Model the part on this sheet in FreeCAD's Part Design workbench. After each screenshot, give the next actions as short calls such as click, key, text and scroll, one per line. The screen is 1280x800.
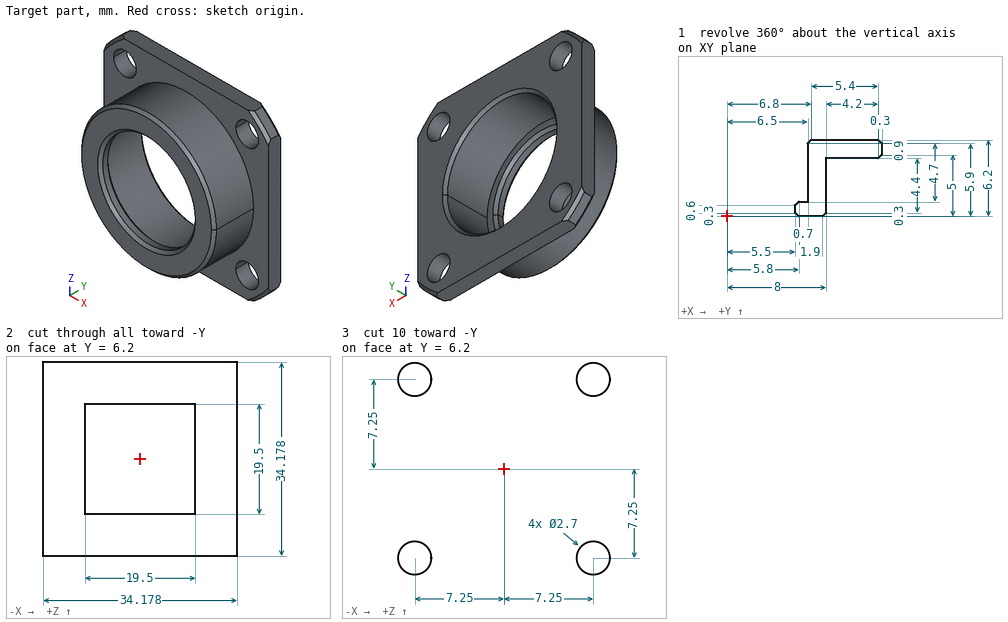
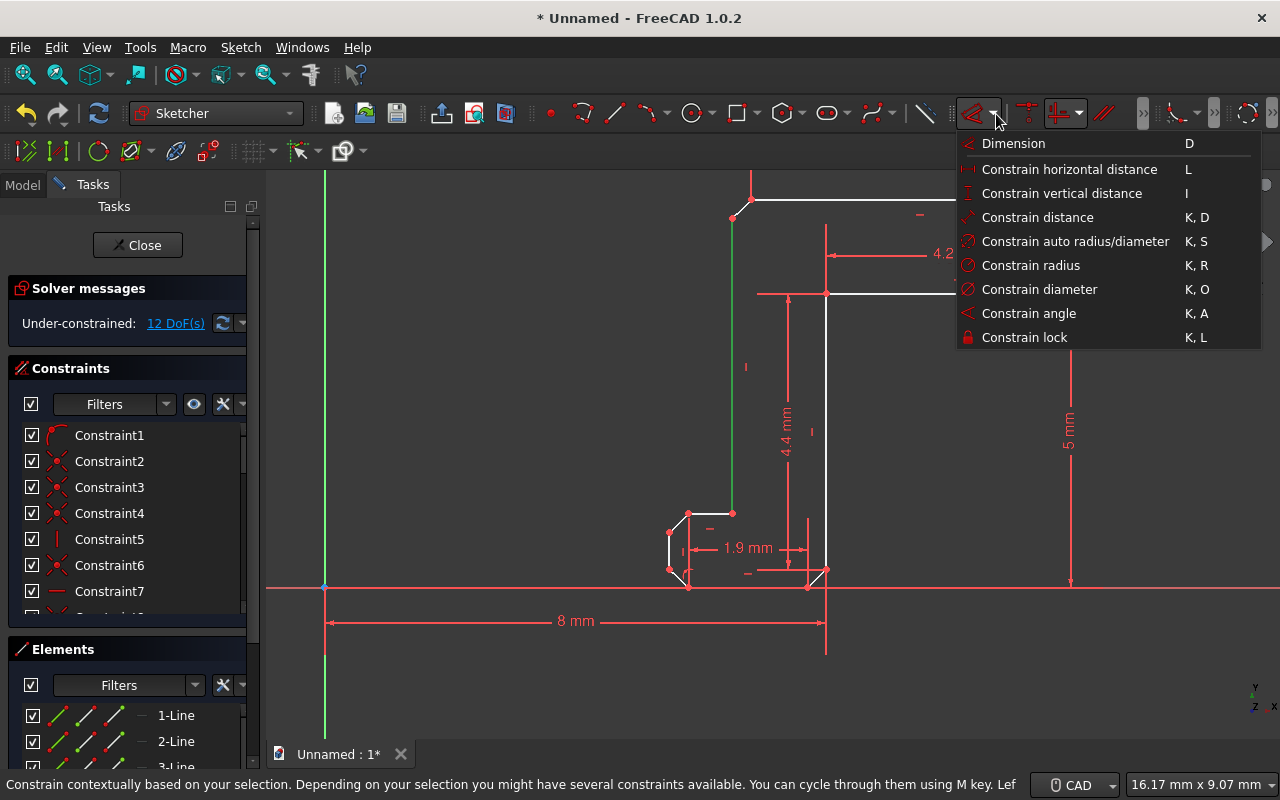
click(1109, 193)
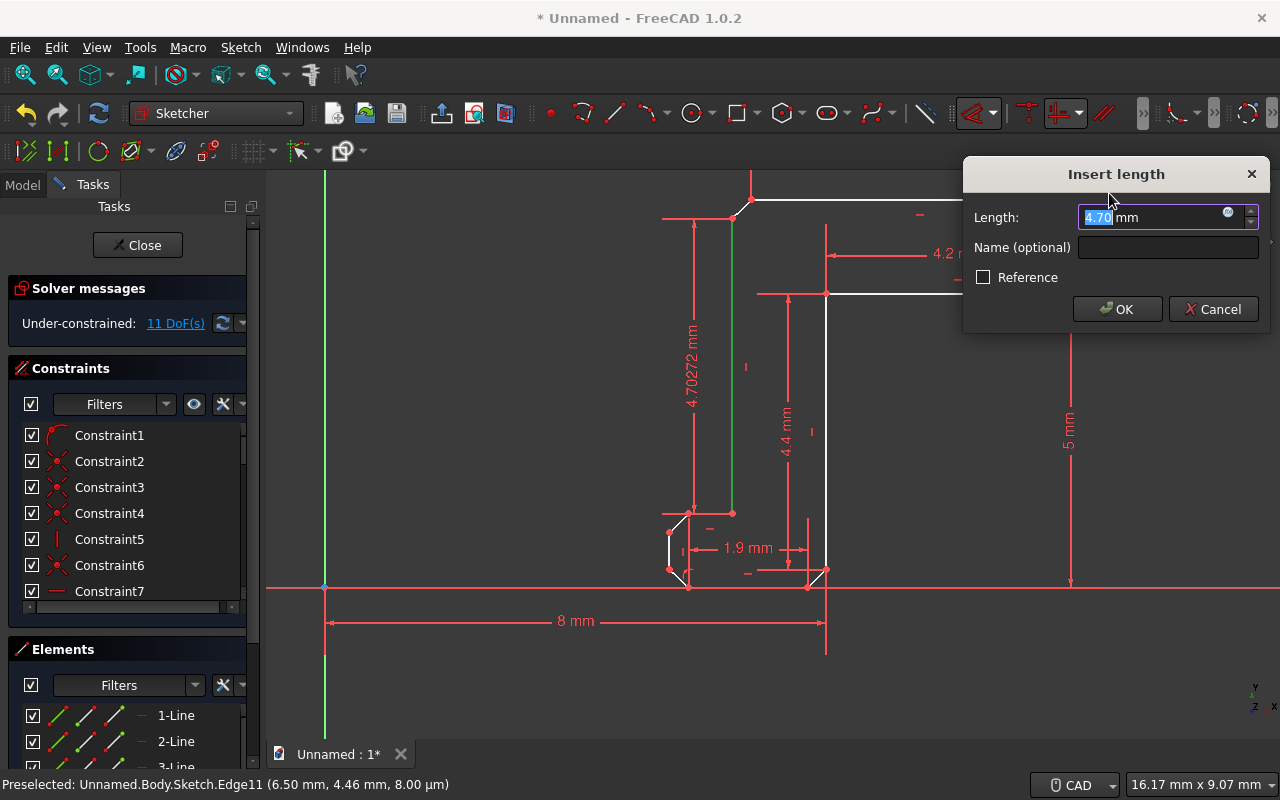
text(4.7)
key(Return)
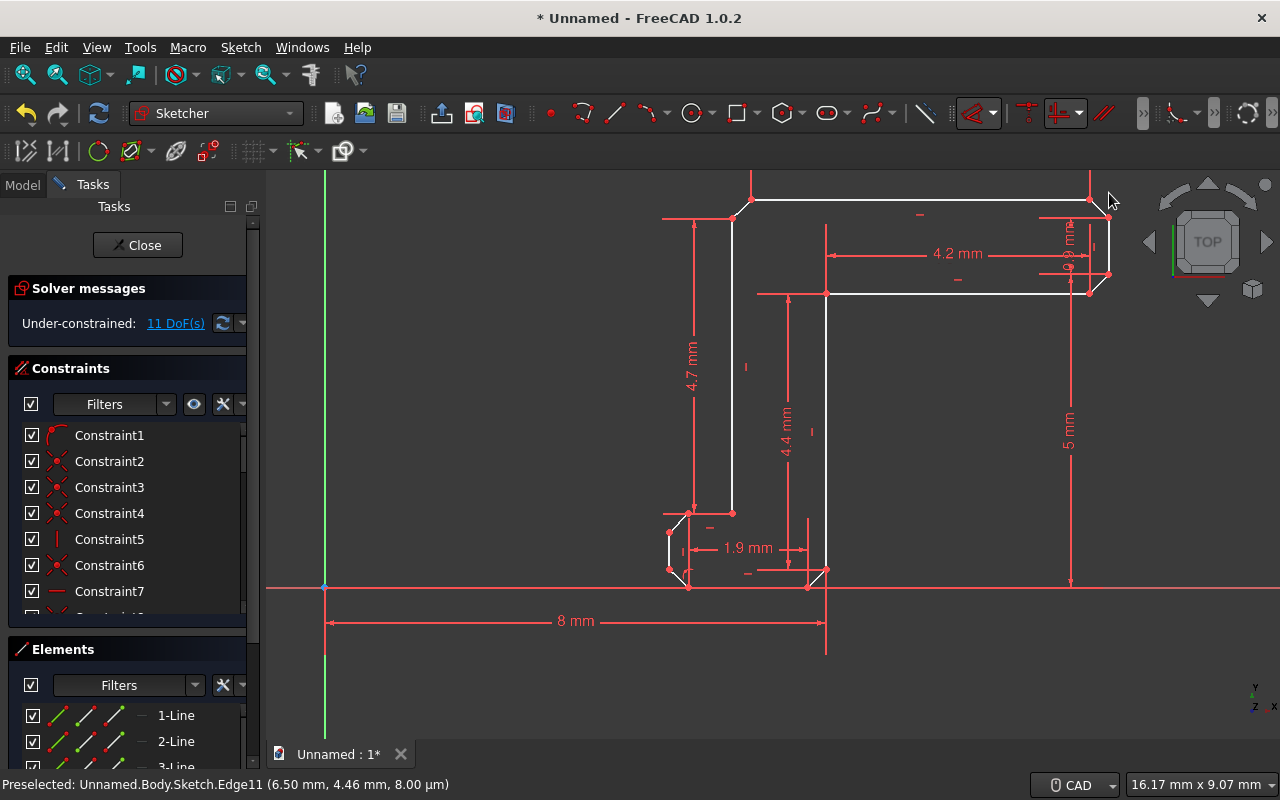
click(719, 514)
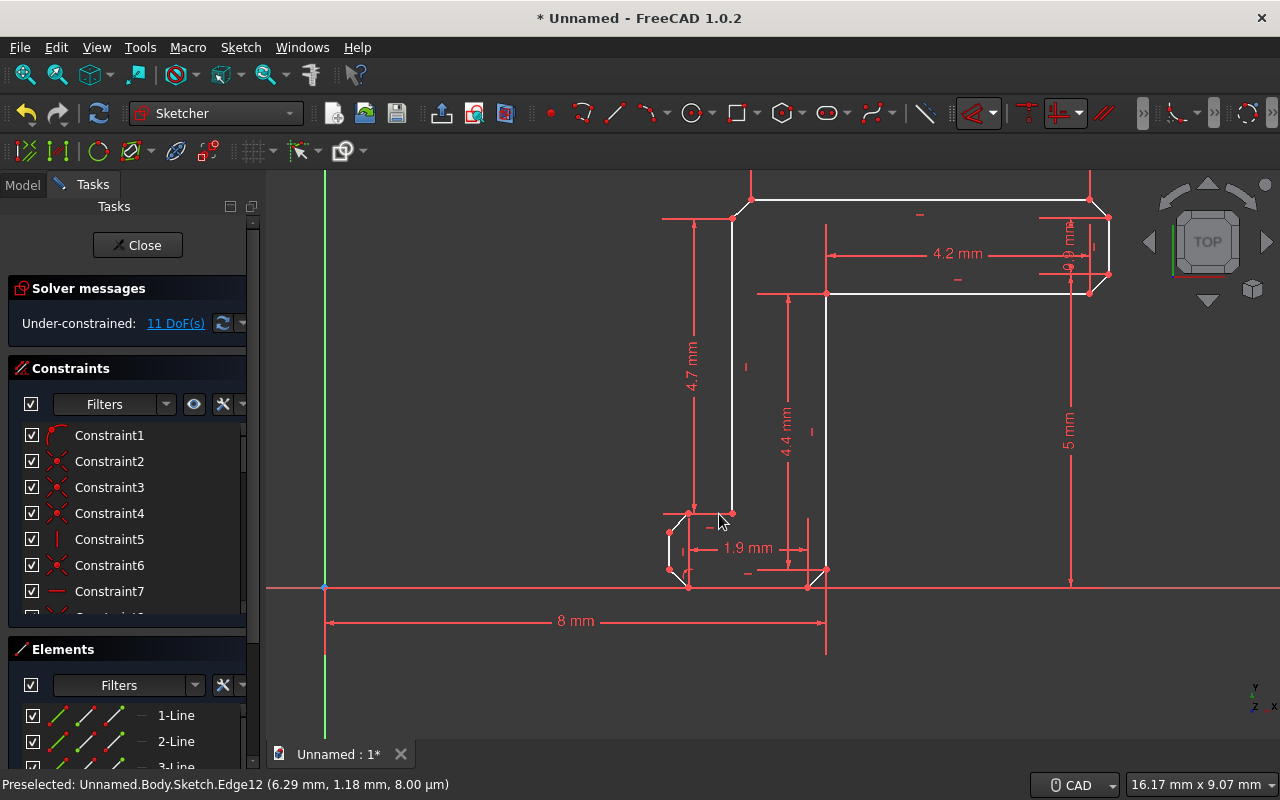
click(996, 114)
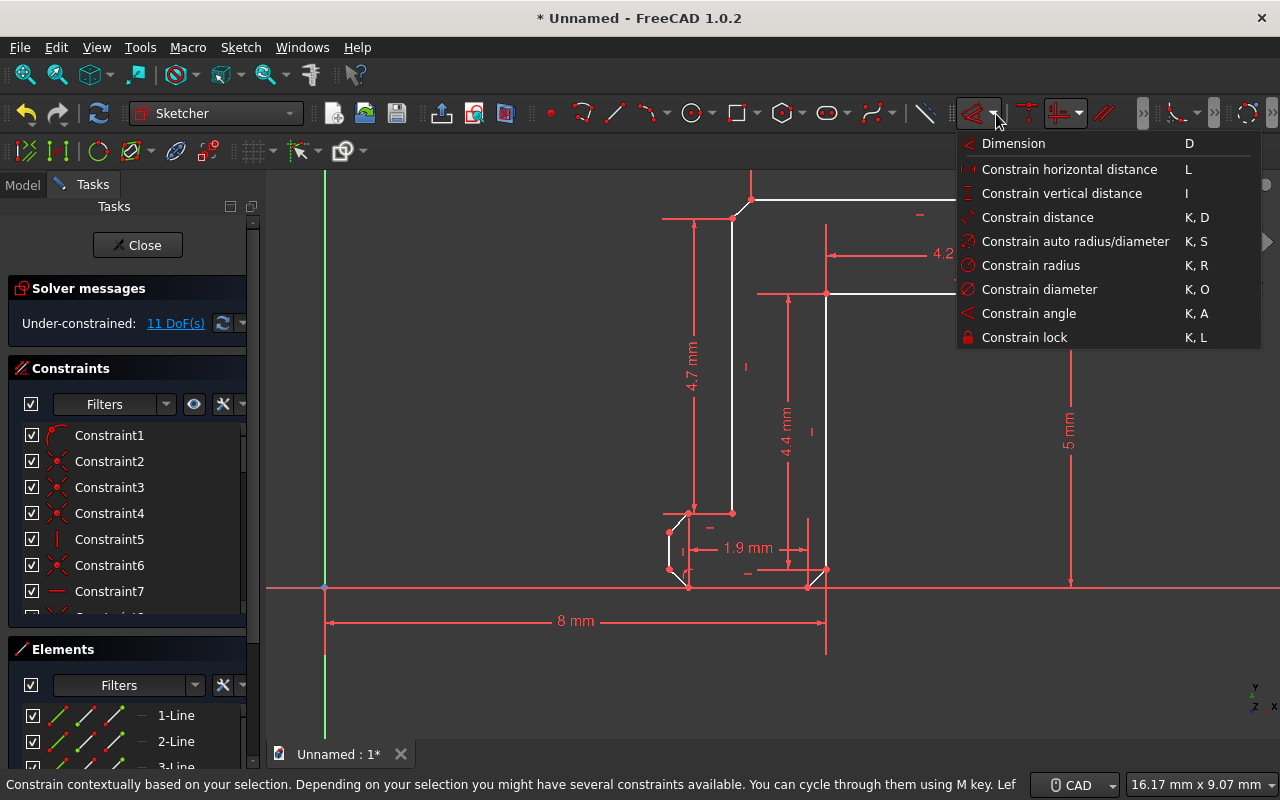
click(1109, 169)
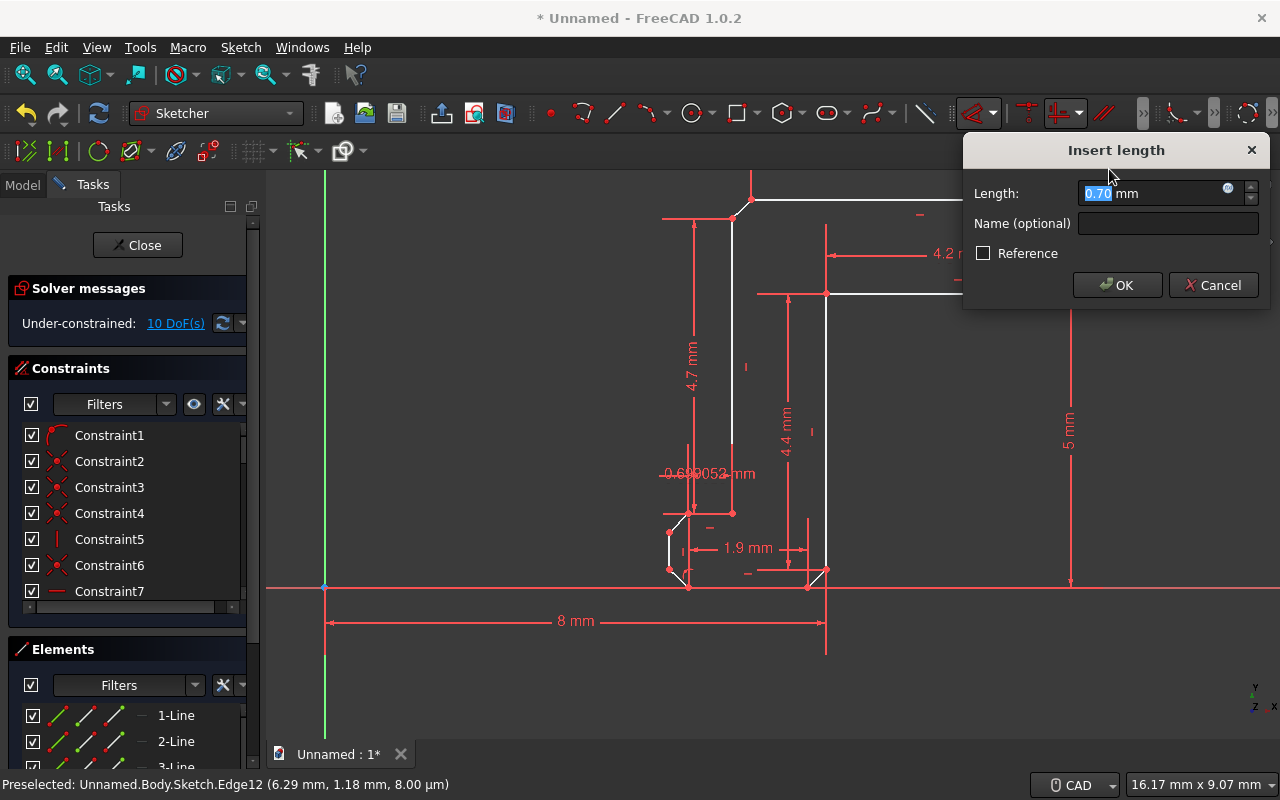
text(0.7)
key(Return)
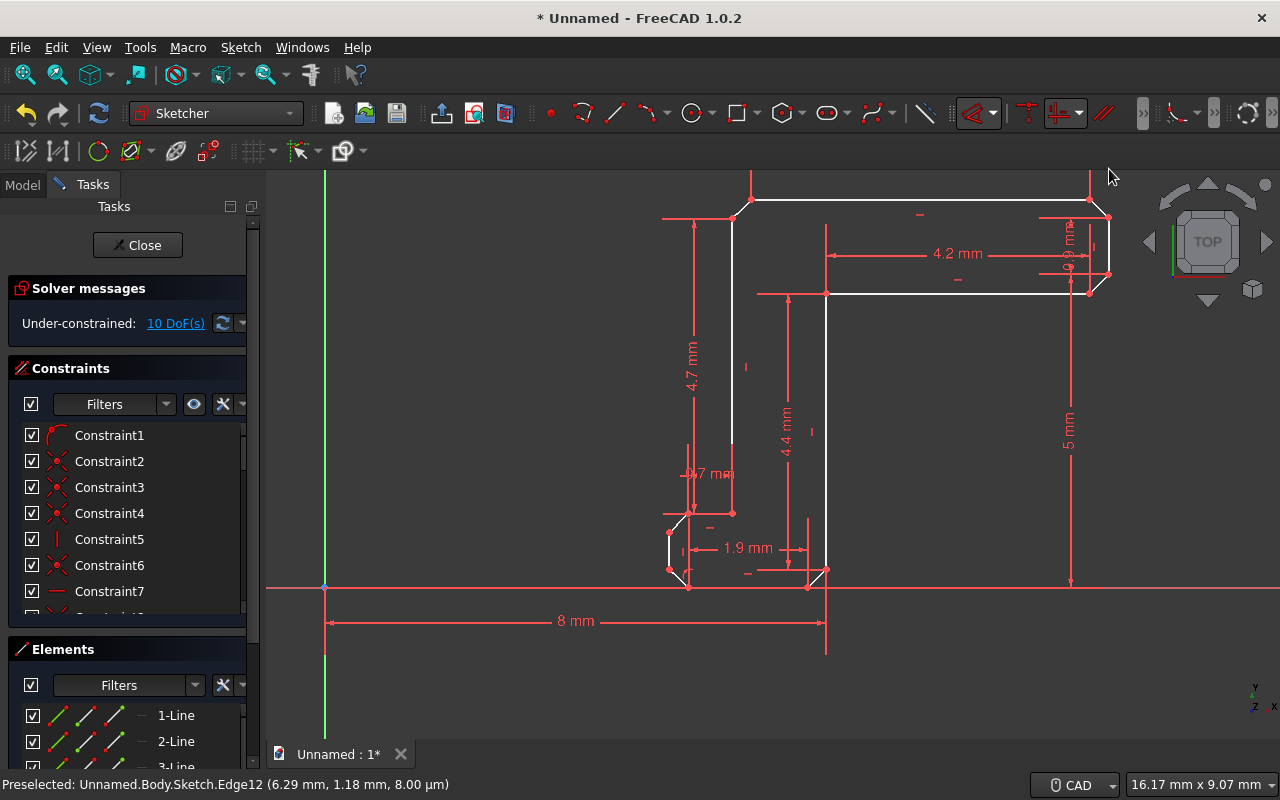
scroll(669, 544, up, 2)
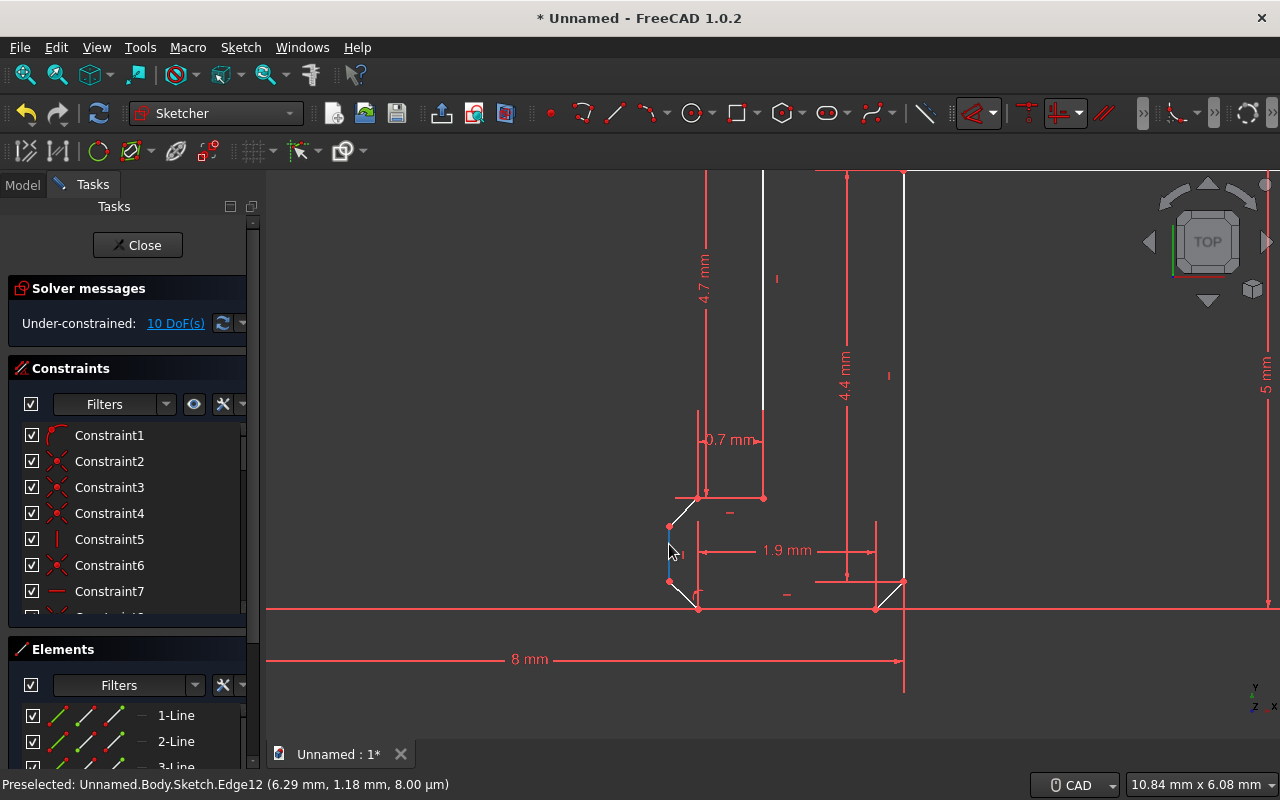
click(669, 543)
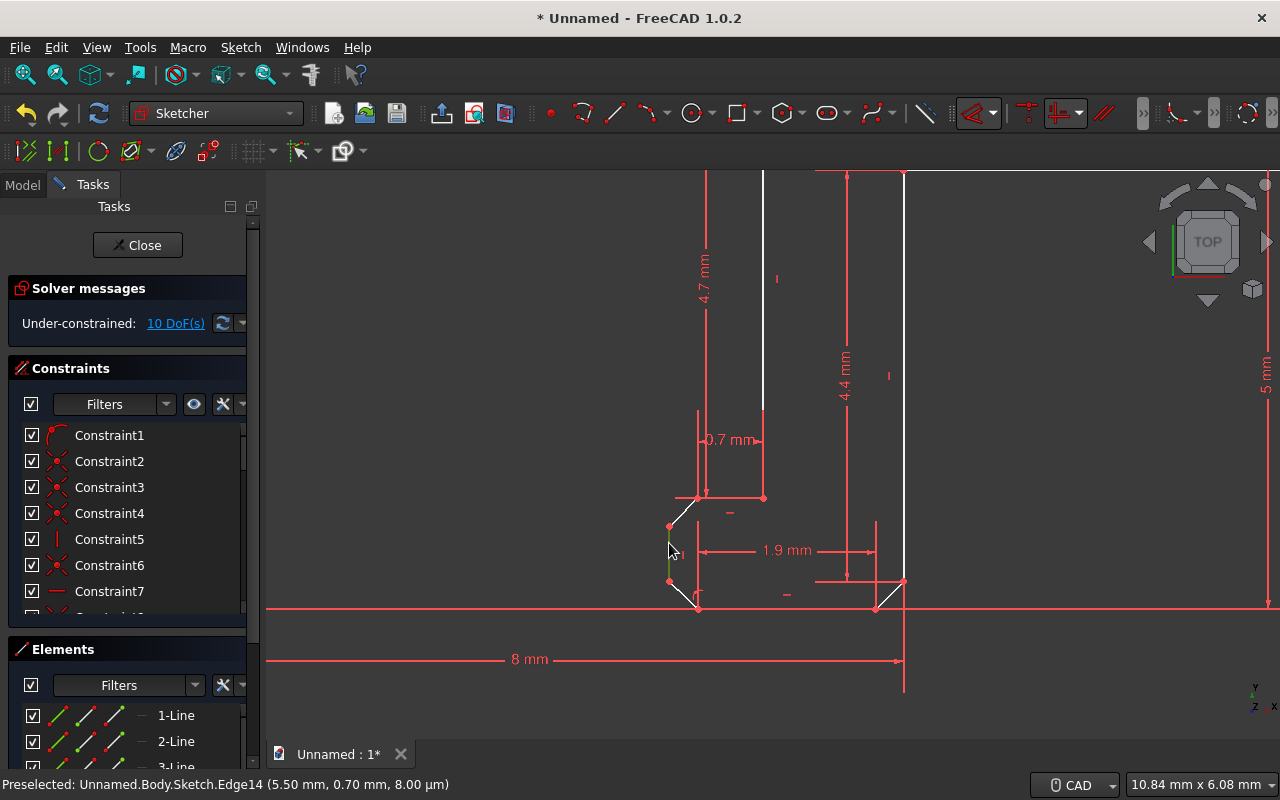
click(996, 114)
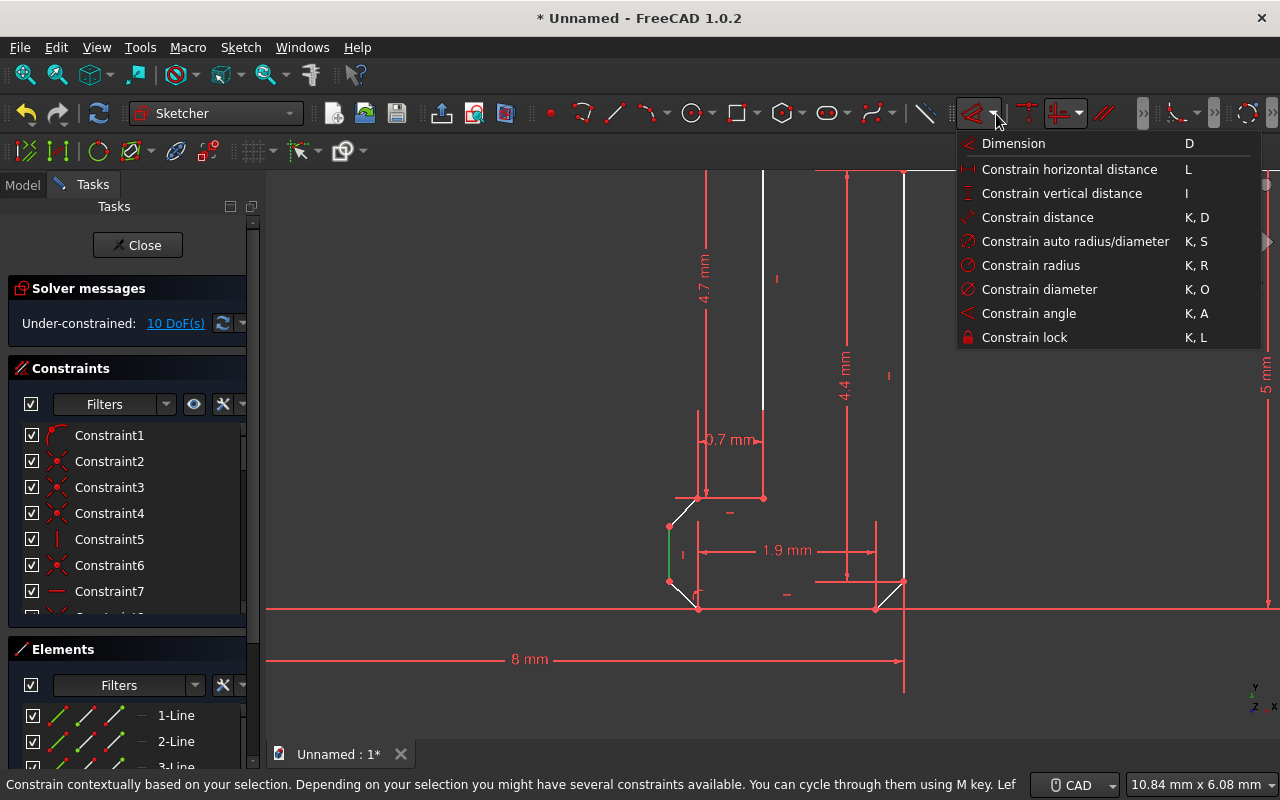
click(1109, 193)